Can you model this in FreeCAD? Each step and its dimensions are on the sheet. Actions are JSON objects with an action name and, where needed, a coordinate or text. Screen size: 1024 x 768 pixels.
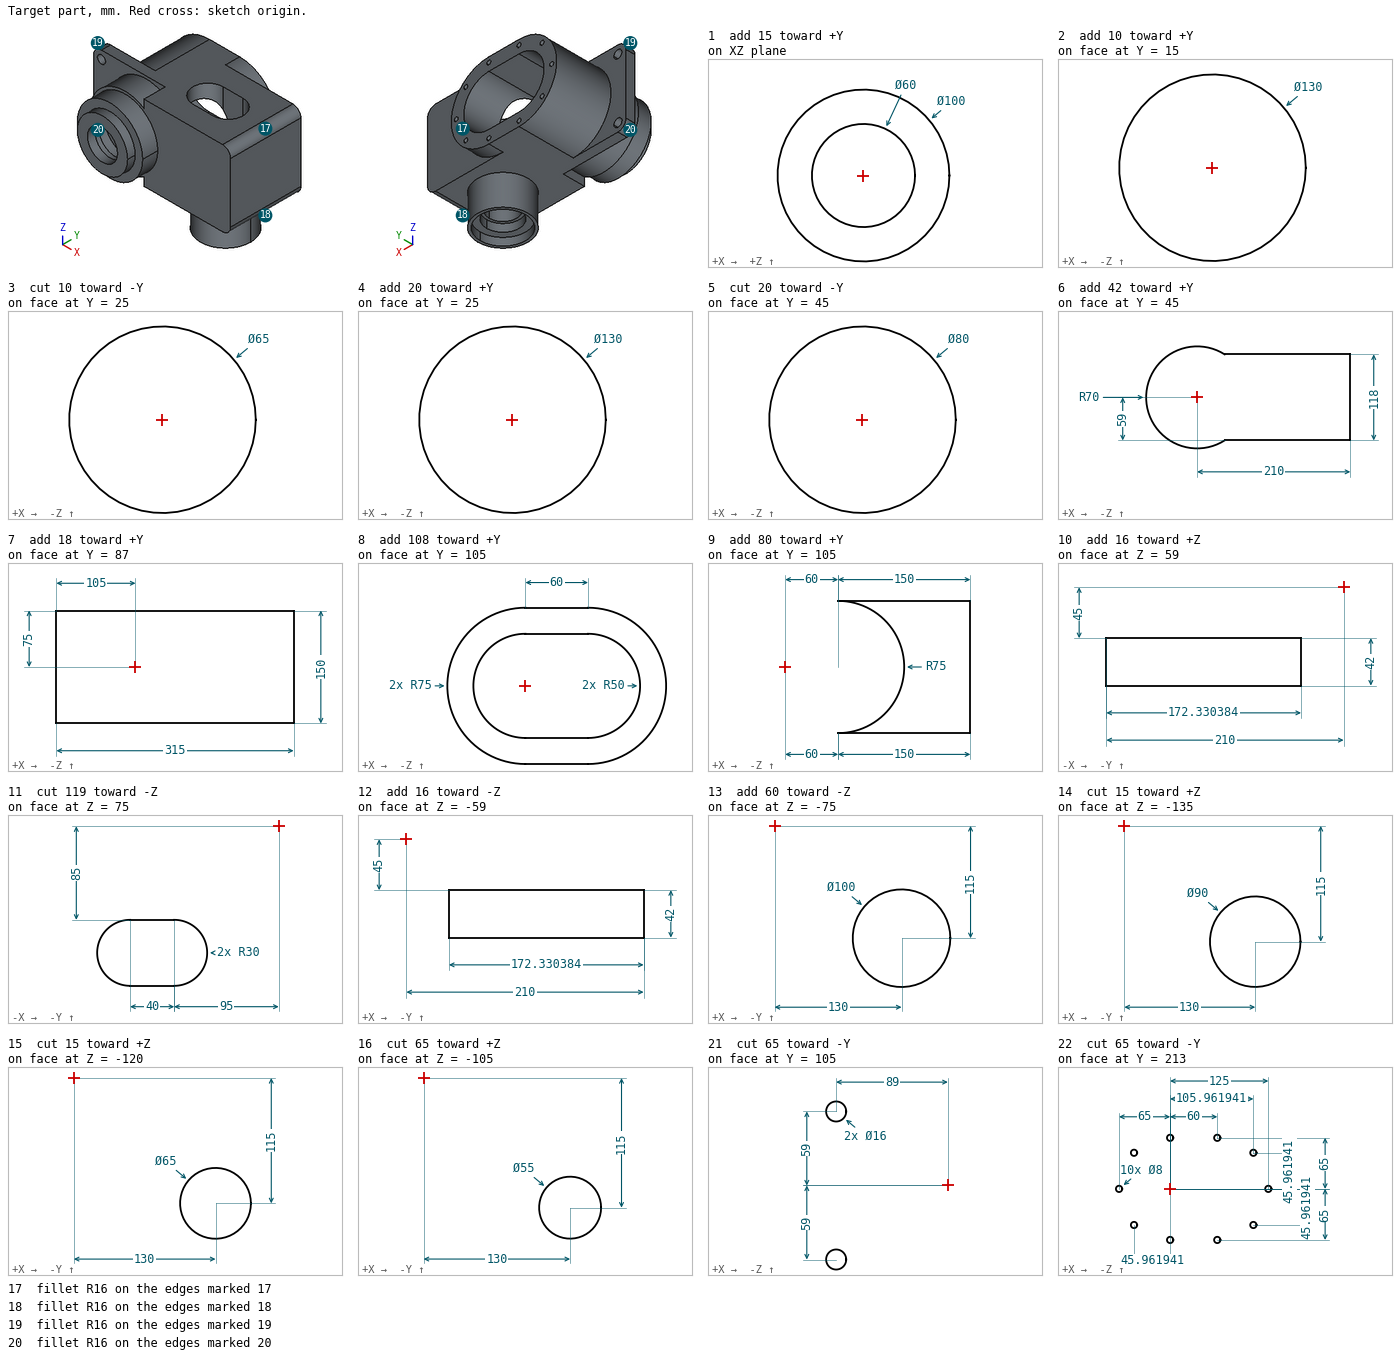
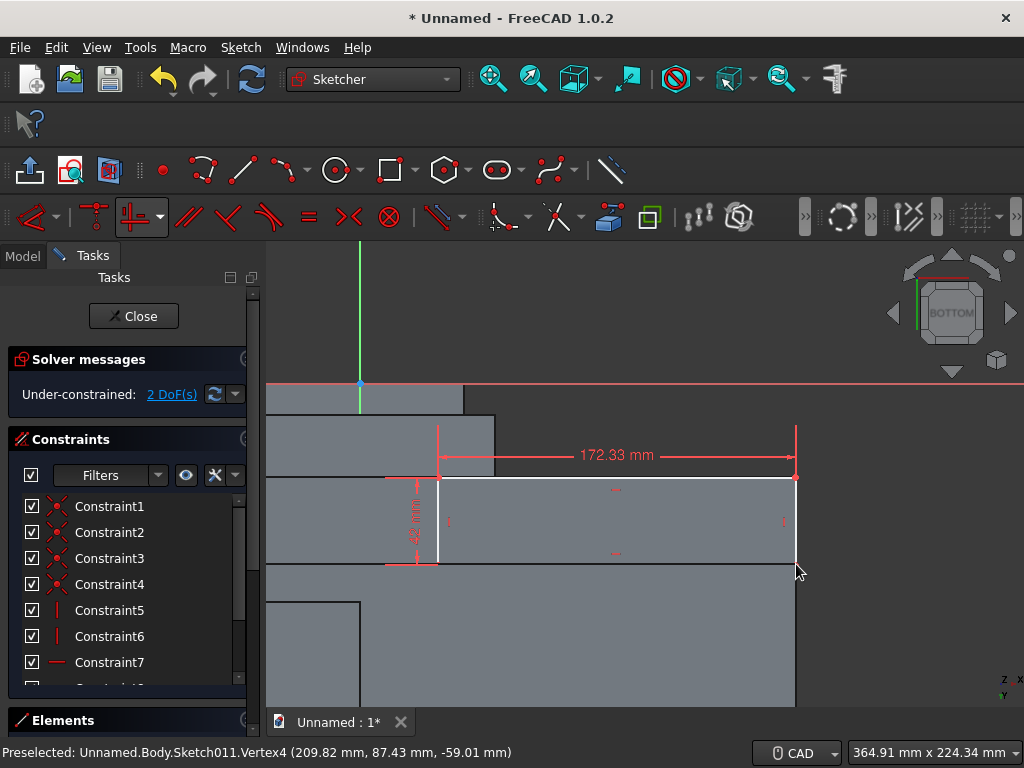
{"action": "left_click", "coordinate": [32, 218]}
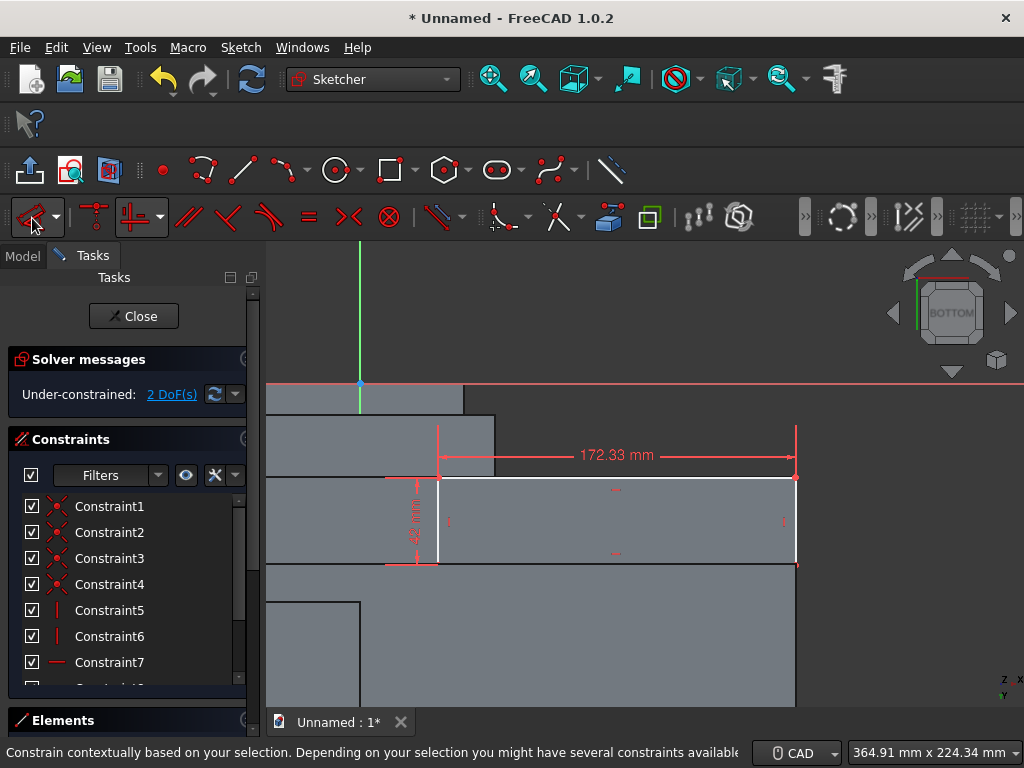
{"action": "left_click", "coordinate": [438, 478]}
{"action": "left_click", "coordinate": [326, 431]}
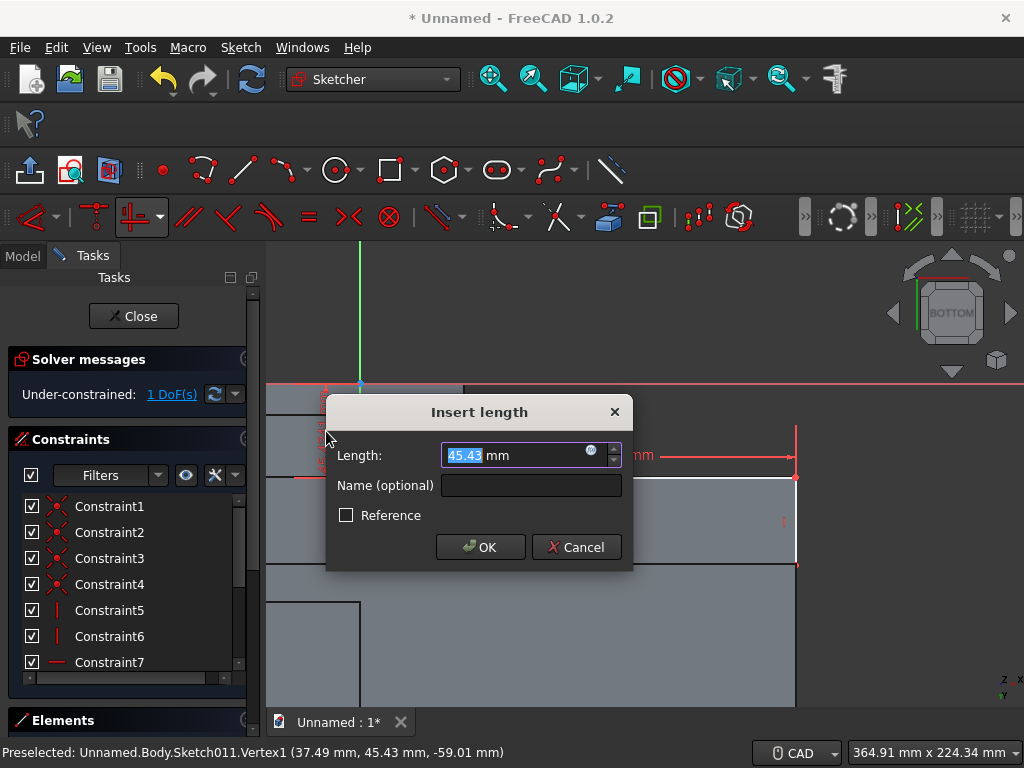
{"action": "type", "text": "45"}
{"action": "key", "text": "Return"}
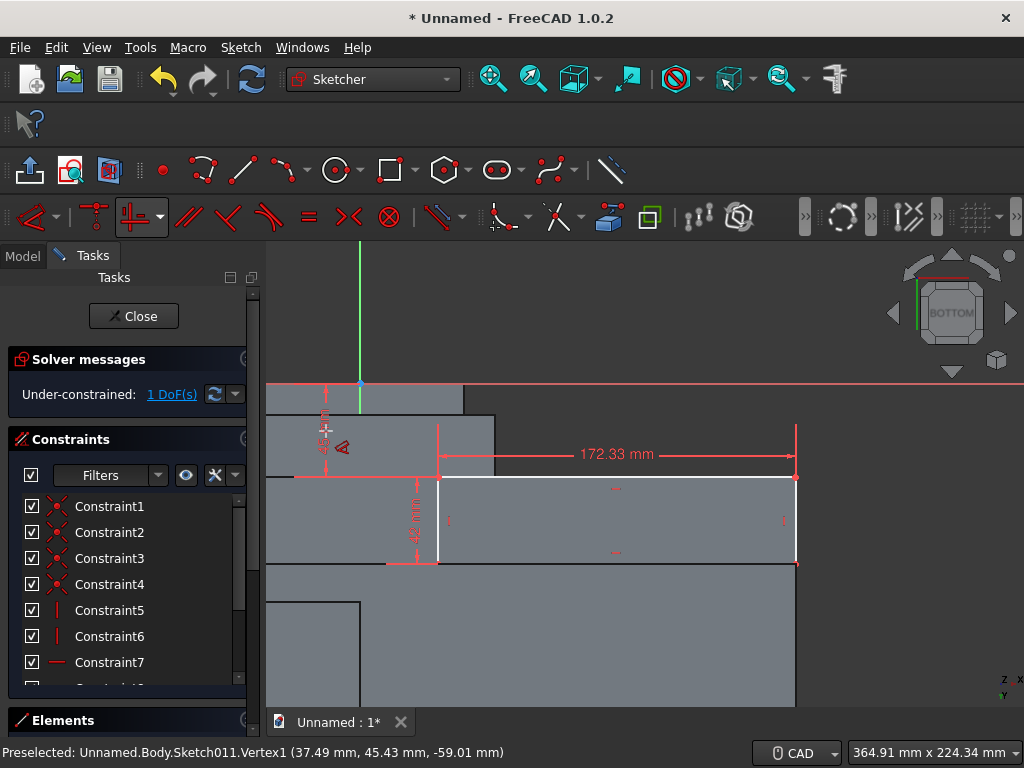
{"action": "left_click", "coordinate": [796, 564]}
{"action": "left_click", "coordinate": [578, 598]}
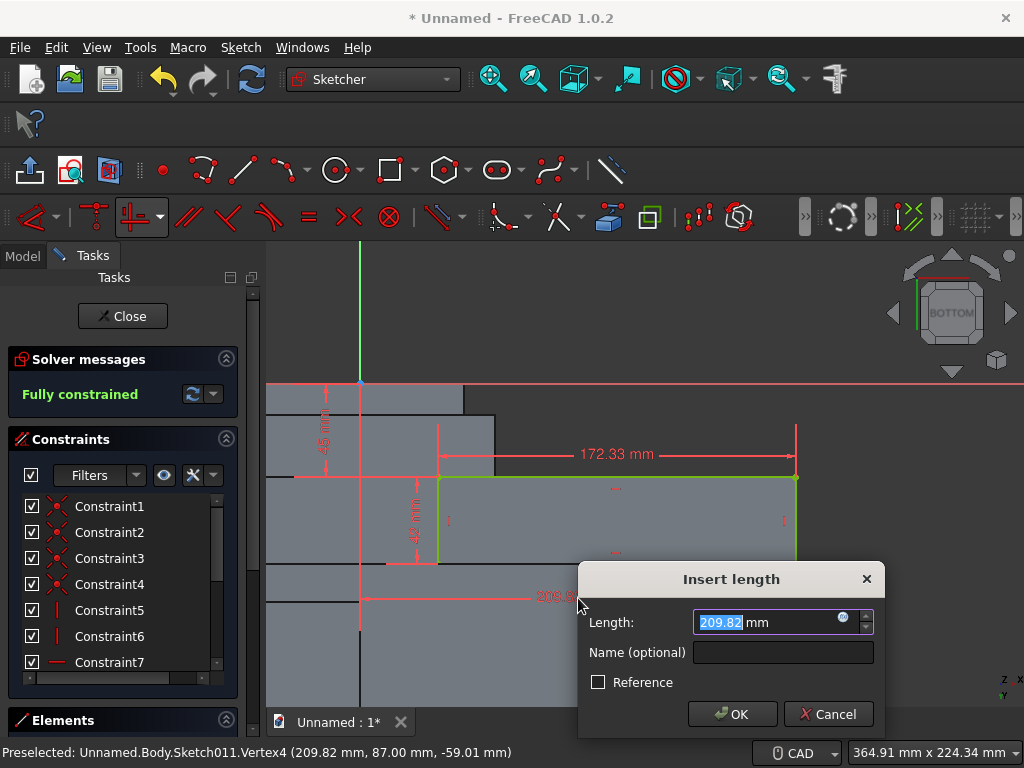
{"action": "type", "text": "210"}
{"action": "key", "text": "Return"}
{"action": "key", "text": "Escape"}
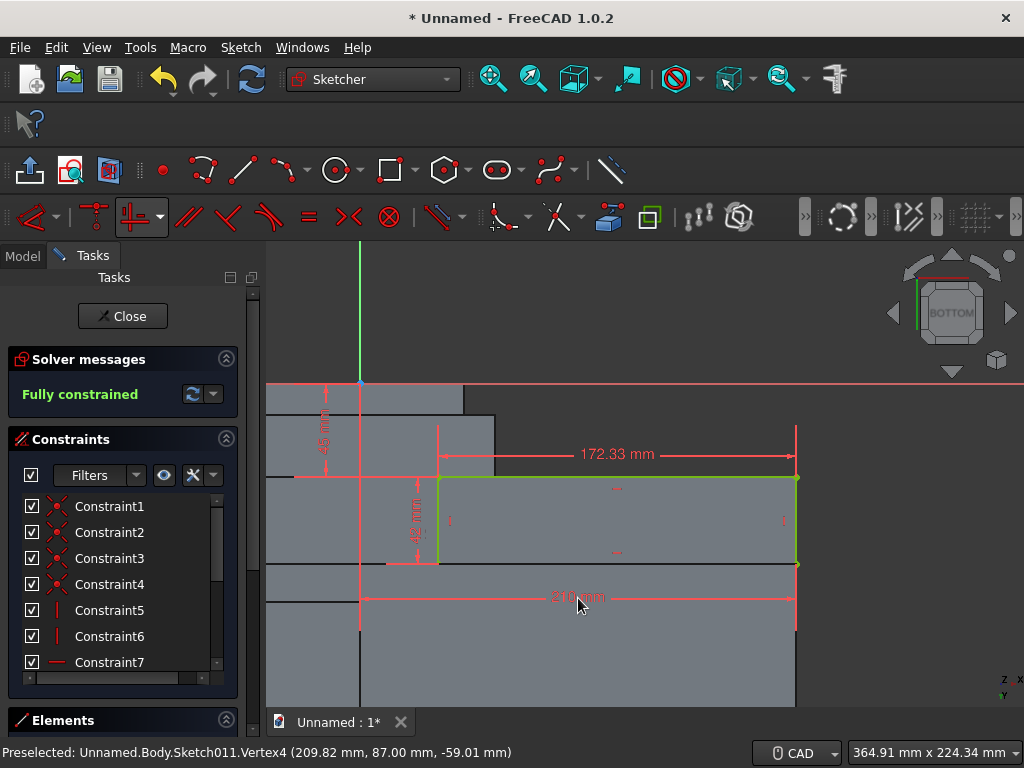
{"action": "left_click", "coordinate": [123, 316]}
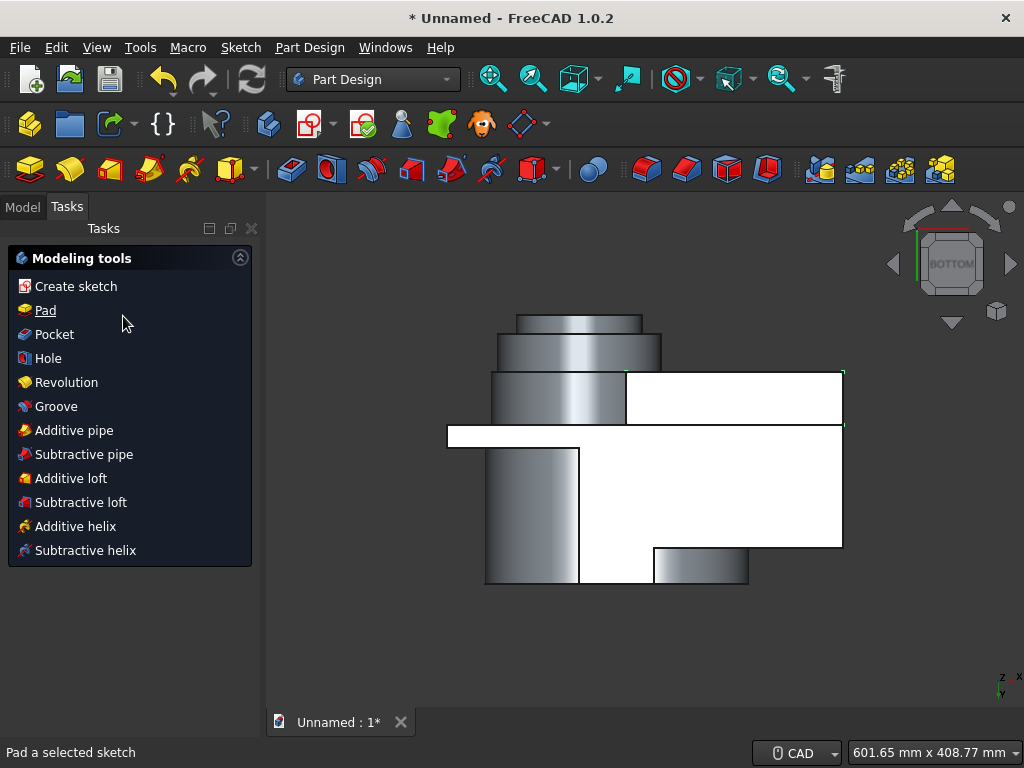
{"action": "left_click", "coordinate": [30, 170]}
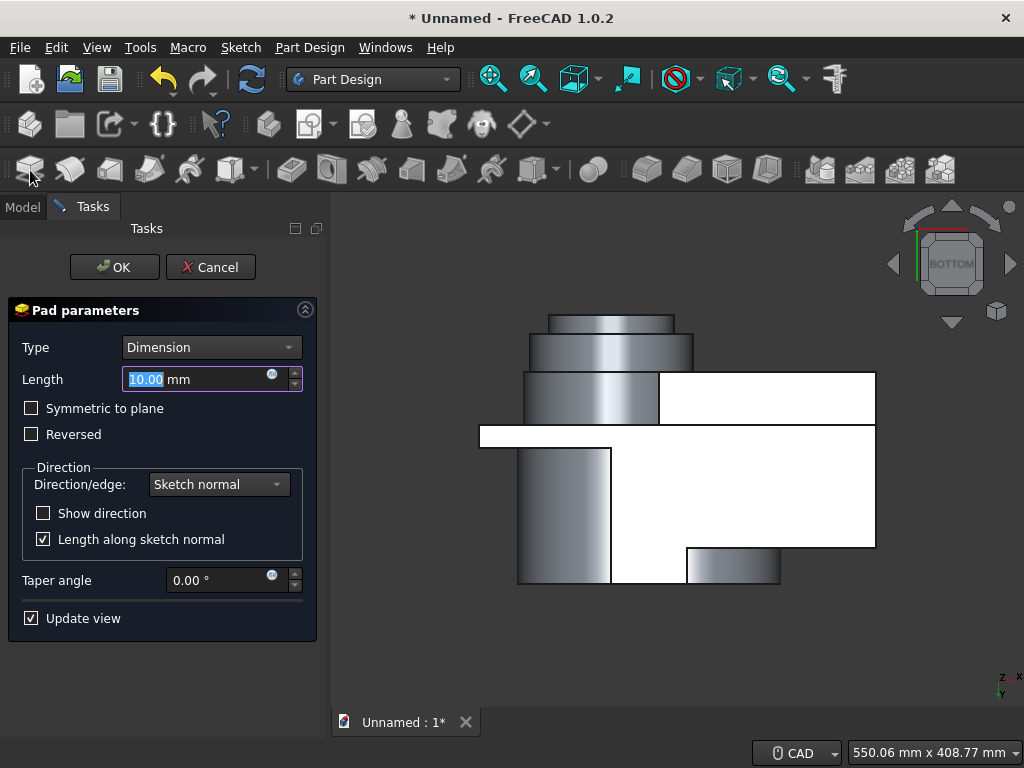
{"action": "type", "text": "16"}
{"action": "key", "text": "Tab"}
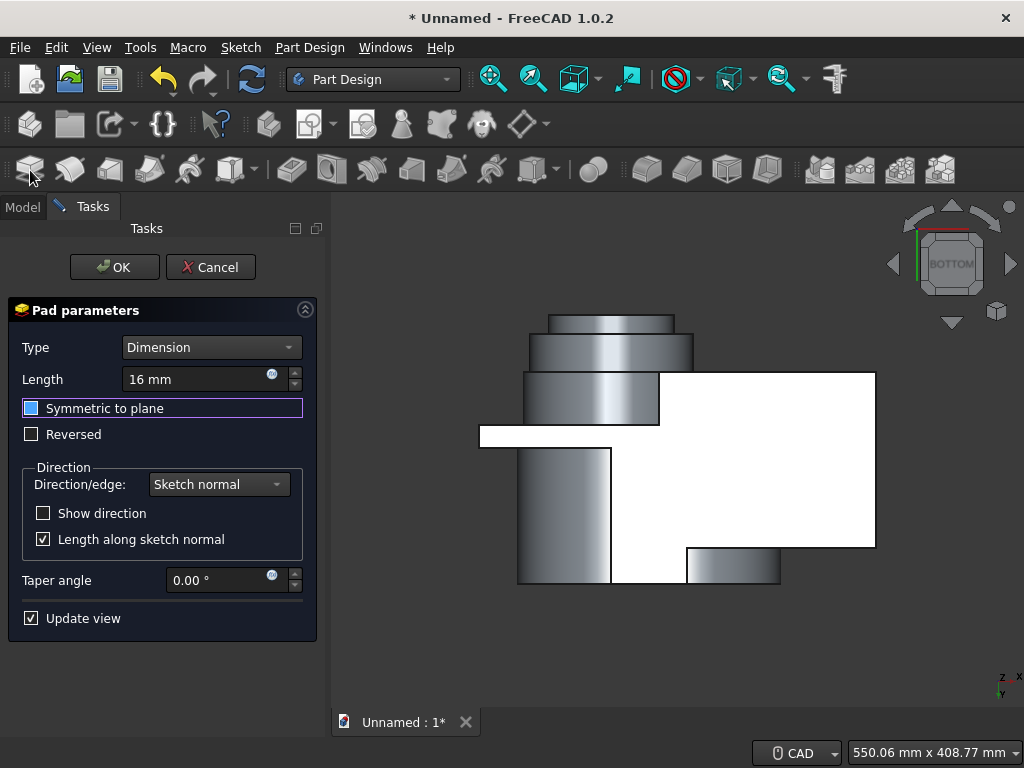
{"action": "left_click", "coordinate": [115, 267]}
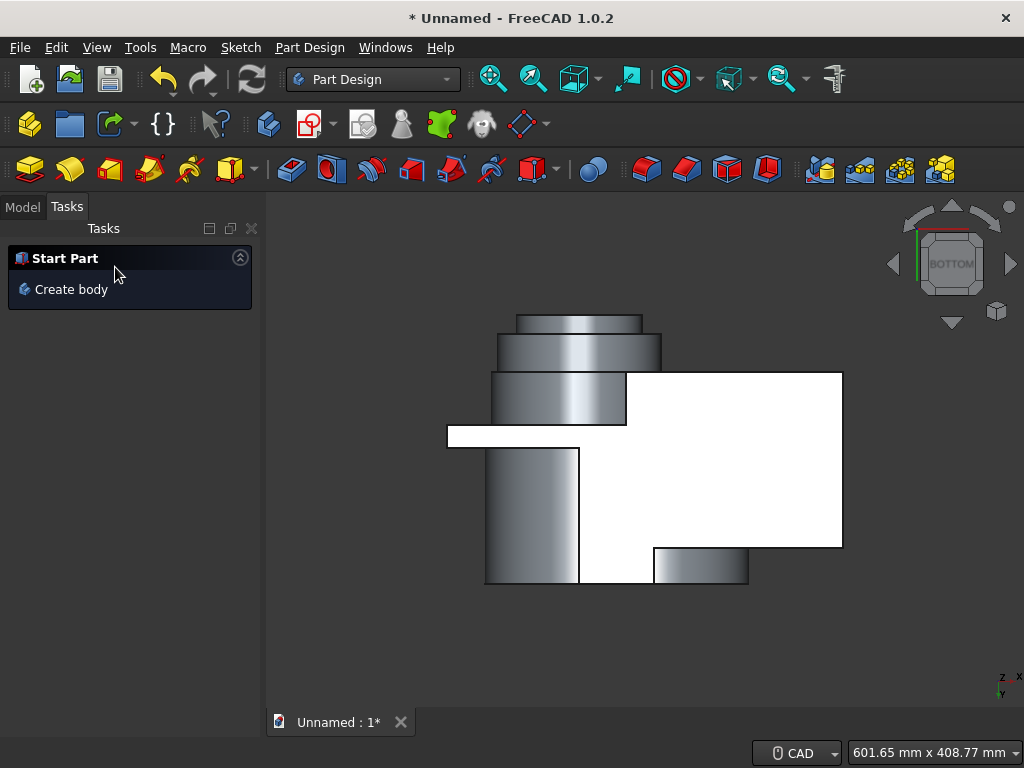
{"action": "left_click", "coordinate": [758, 447]}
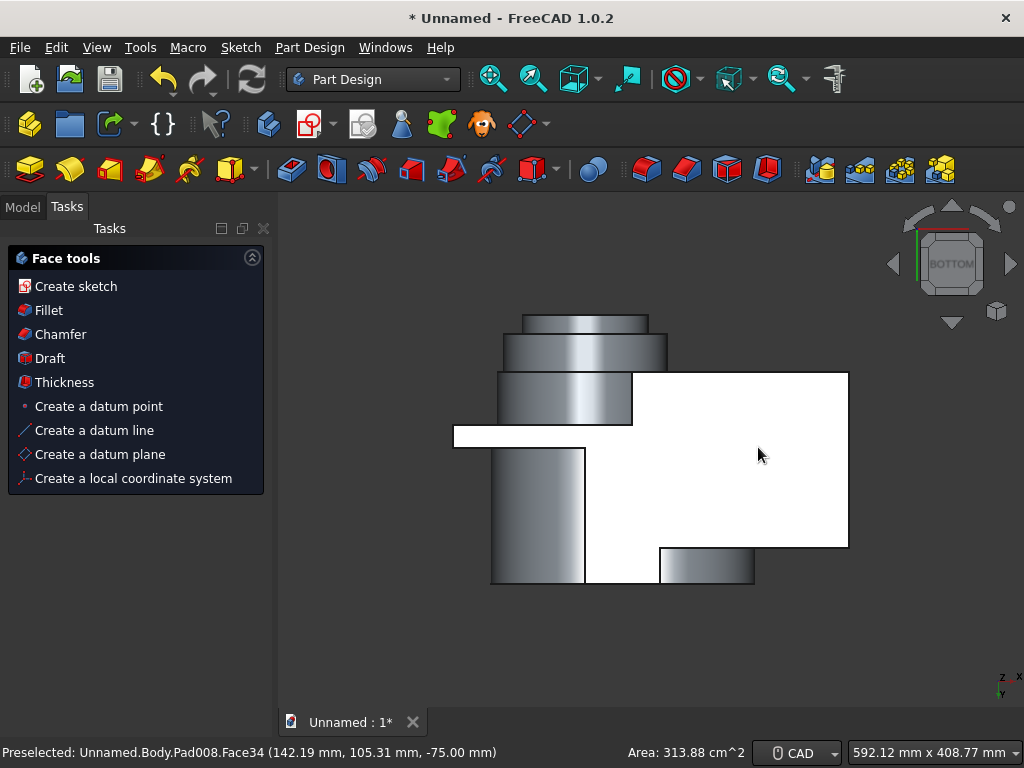
{"action": "left_click", "coordinate": [310, 124]}